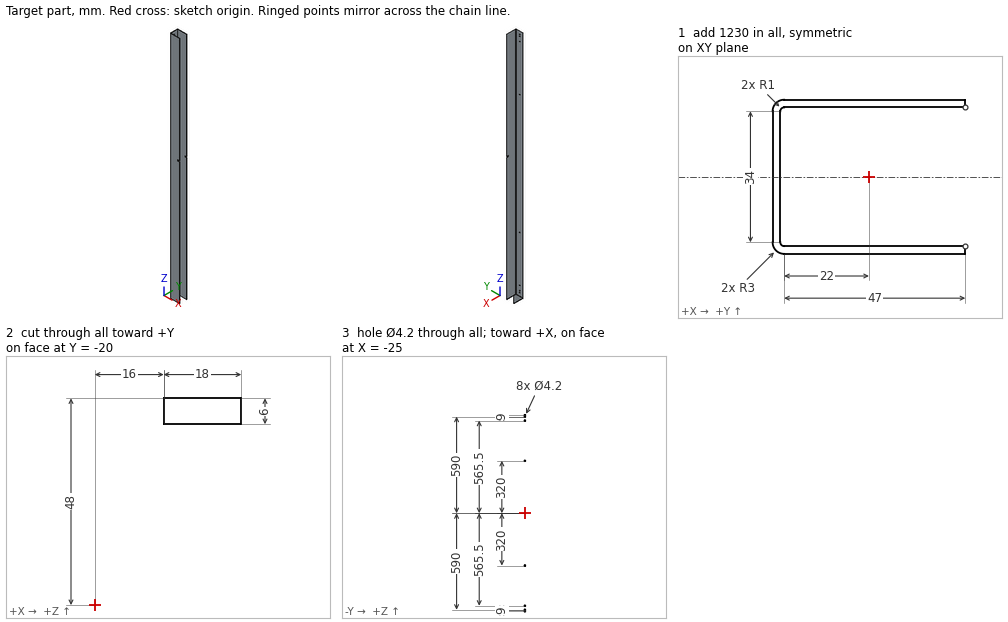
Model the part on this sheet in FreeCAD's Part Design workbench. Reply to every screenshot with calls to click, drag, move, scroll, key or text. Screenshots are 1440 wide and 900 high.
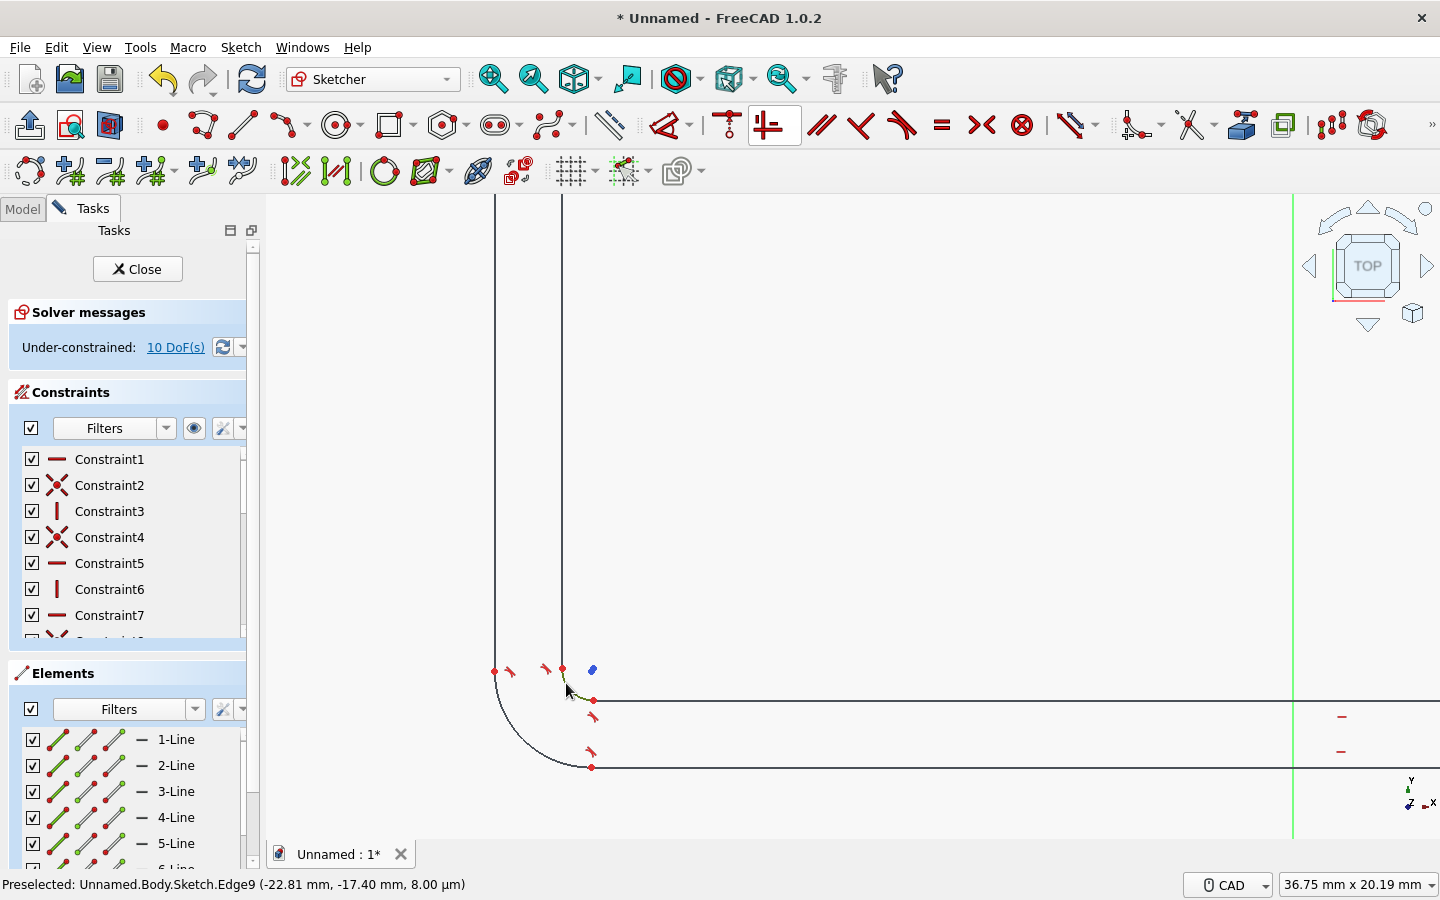
click(505, 715)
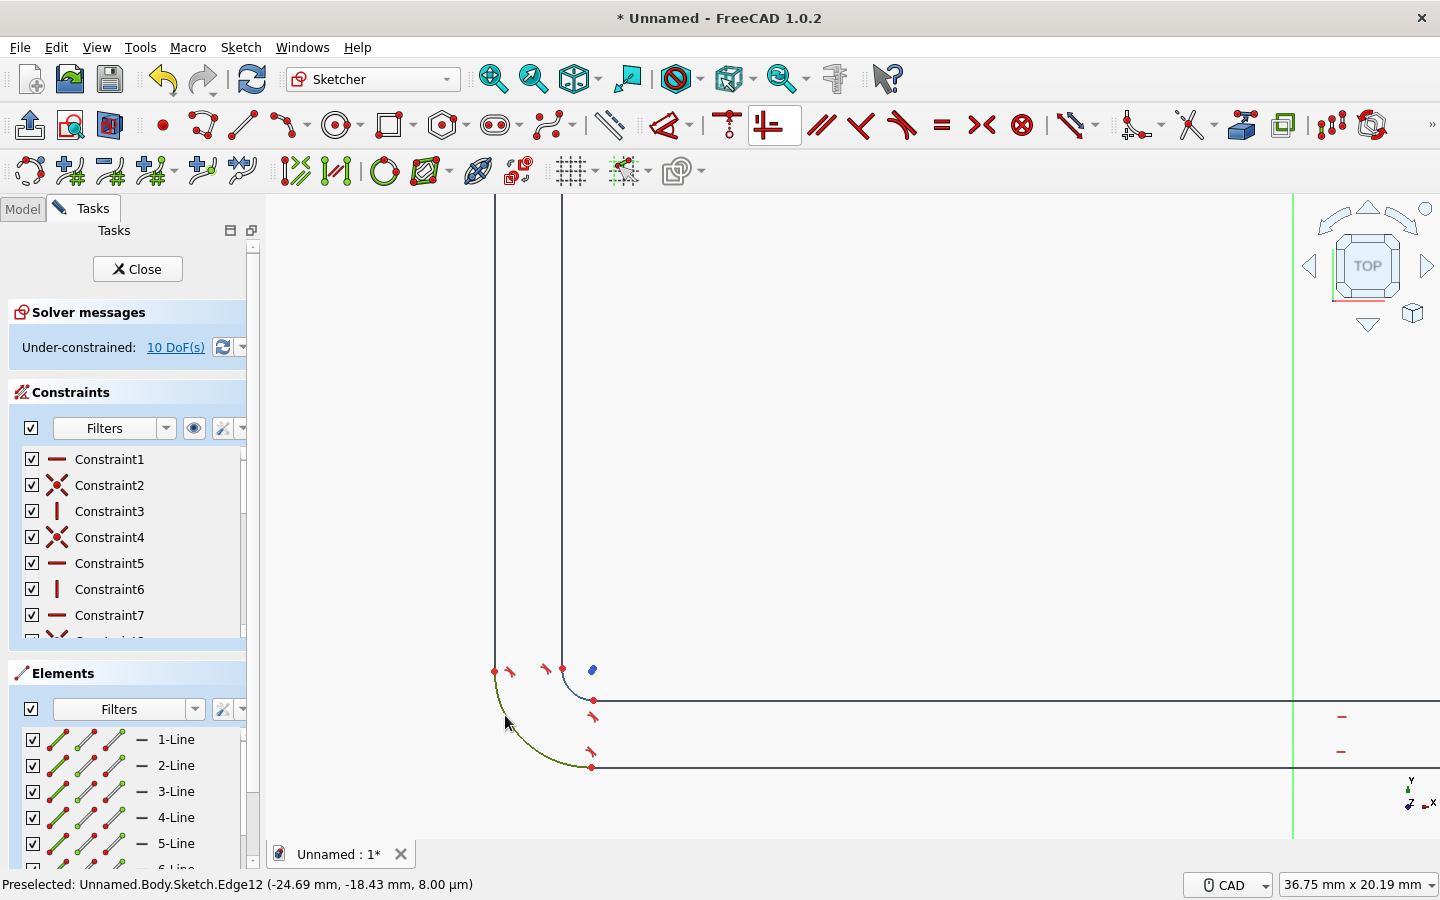
click(728, 126)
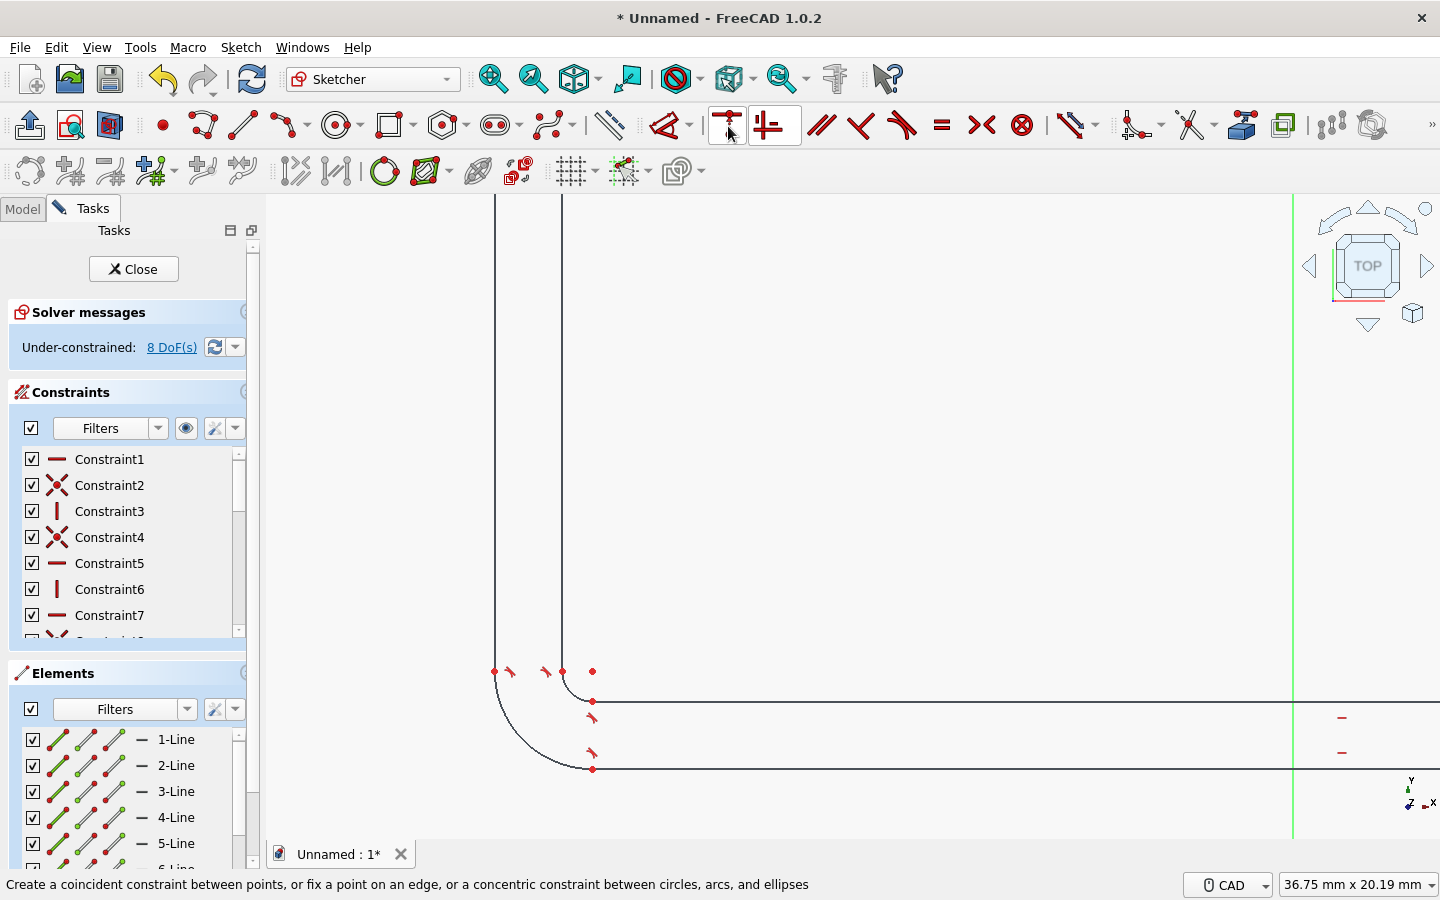
click(566, 685)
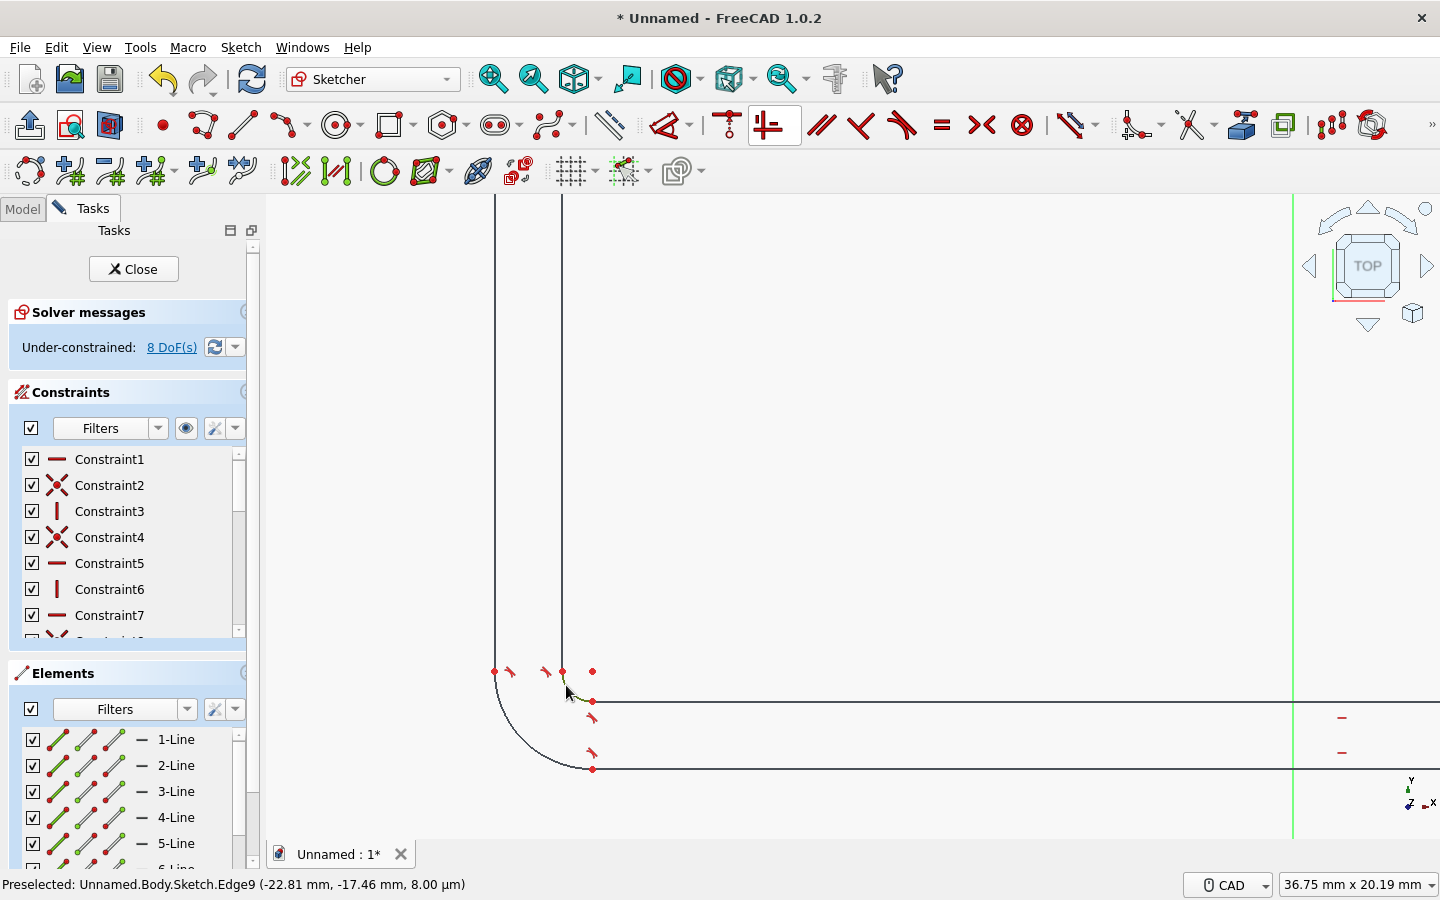
scroll(565, 686, down, 6)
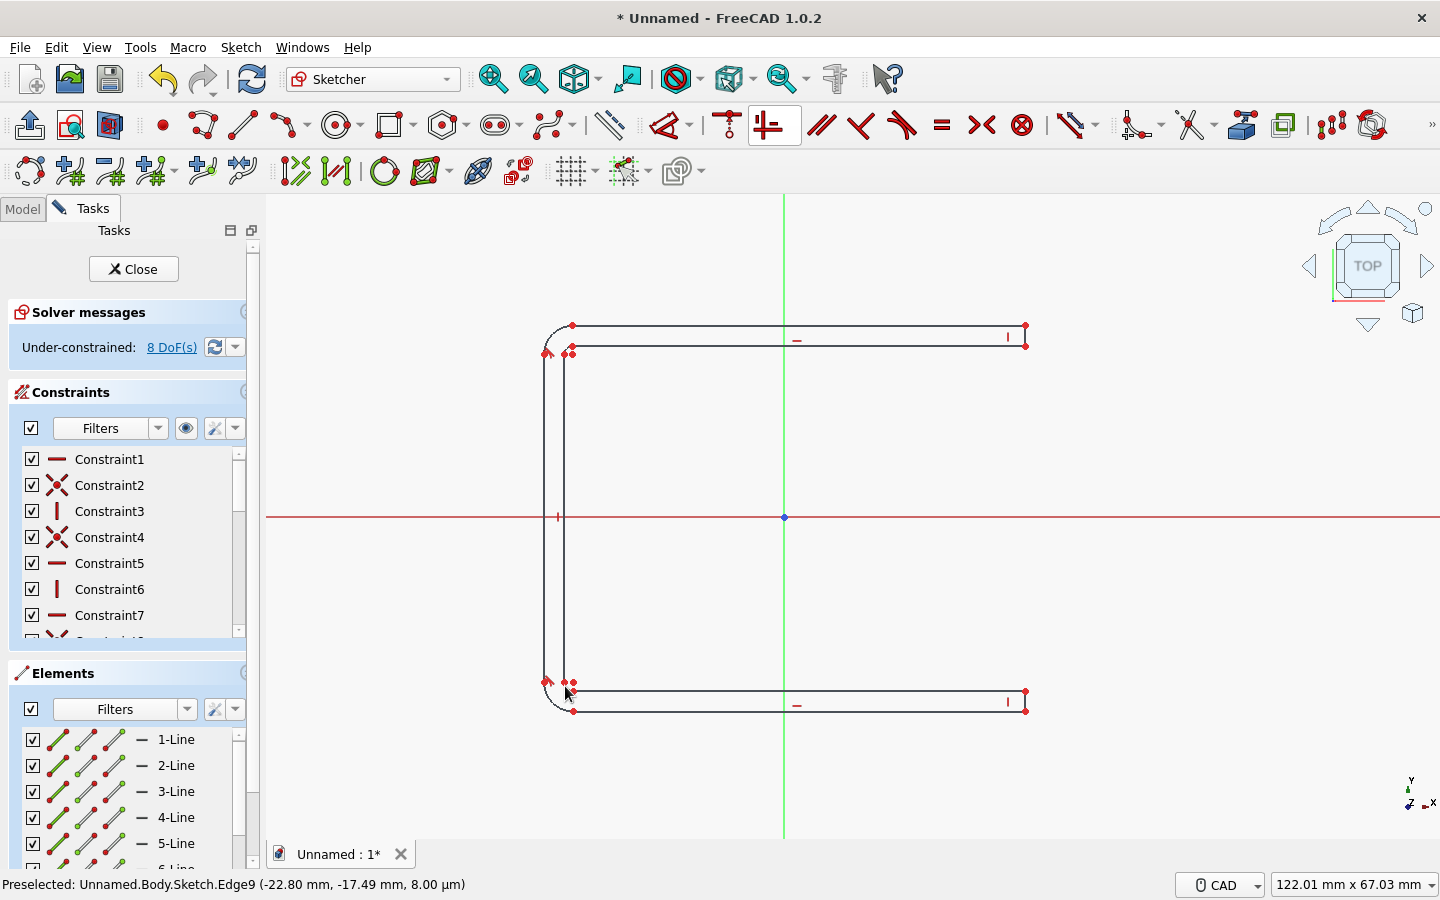
scroll(569, 347, up, 7)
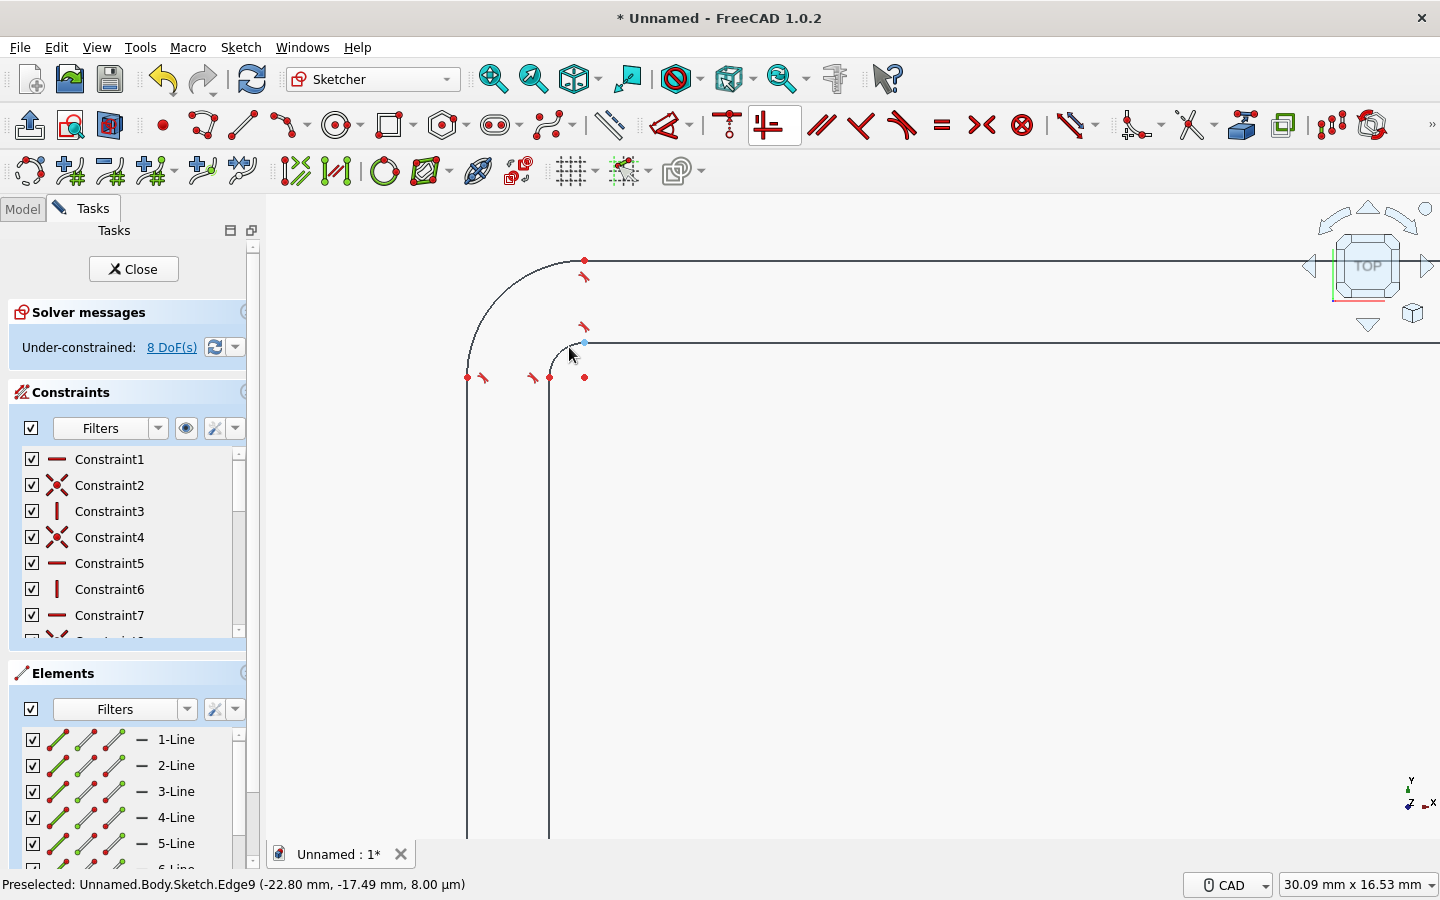
click(568, 347)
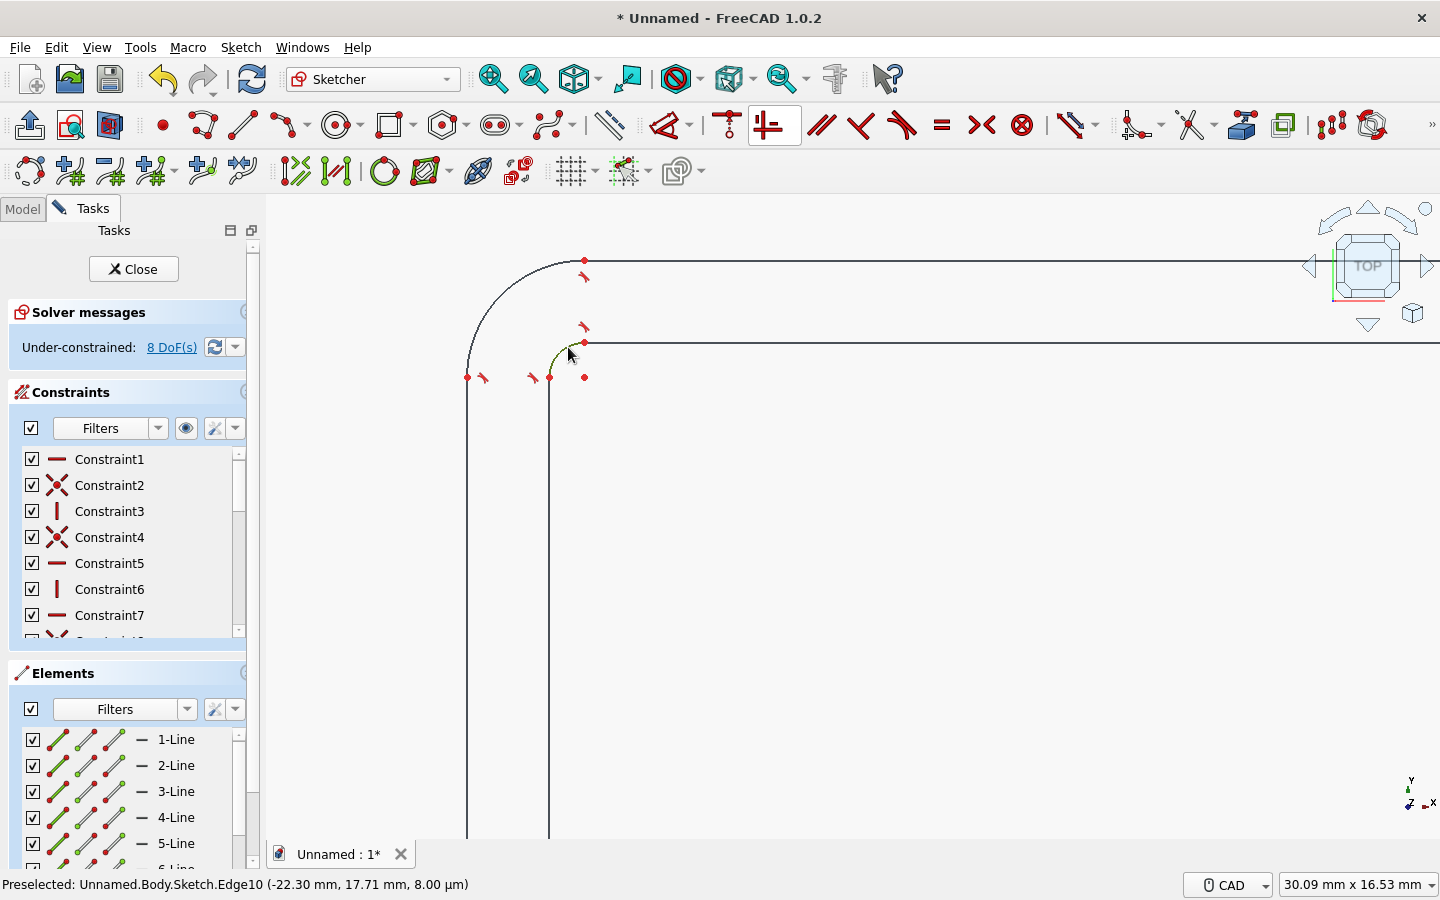
key(e)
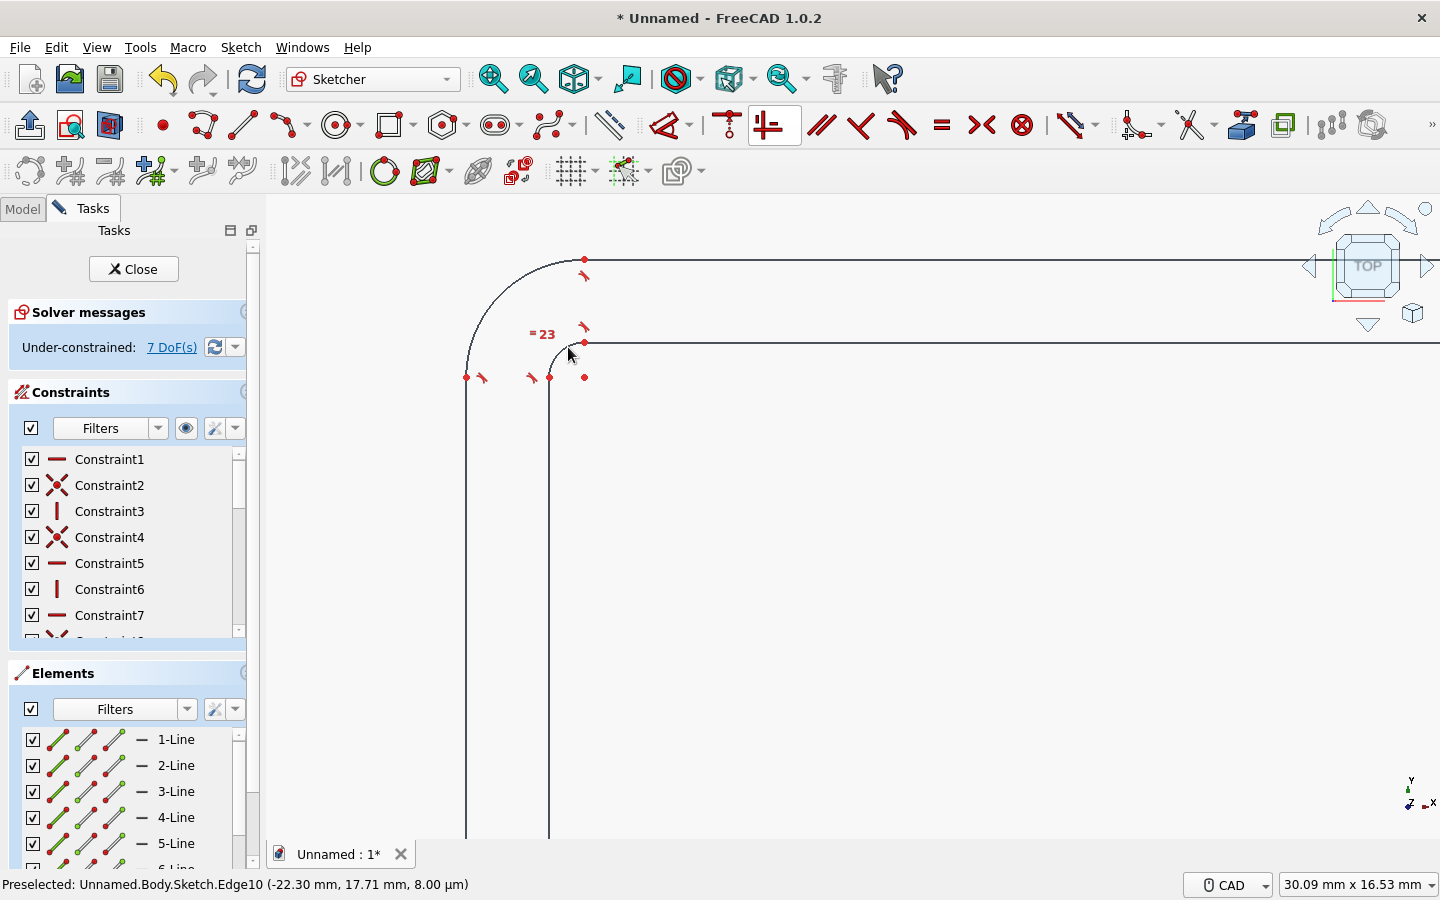
scroll(569, 346, down, 7)